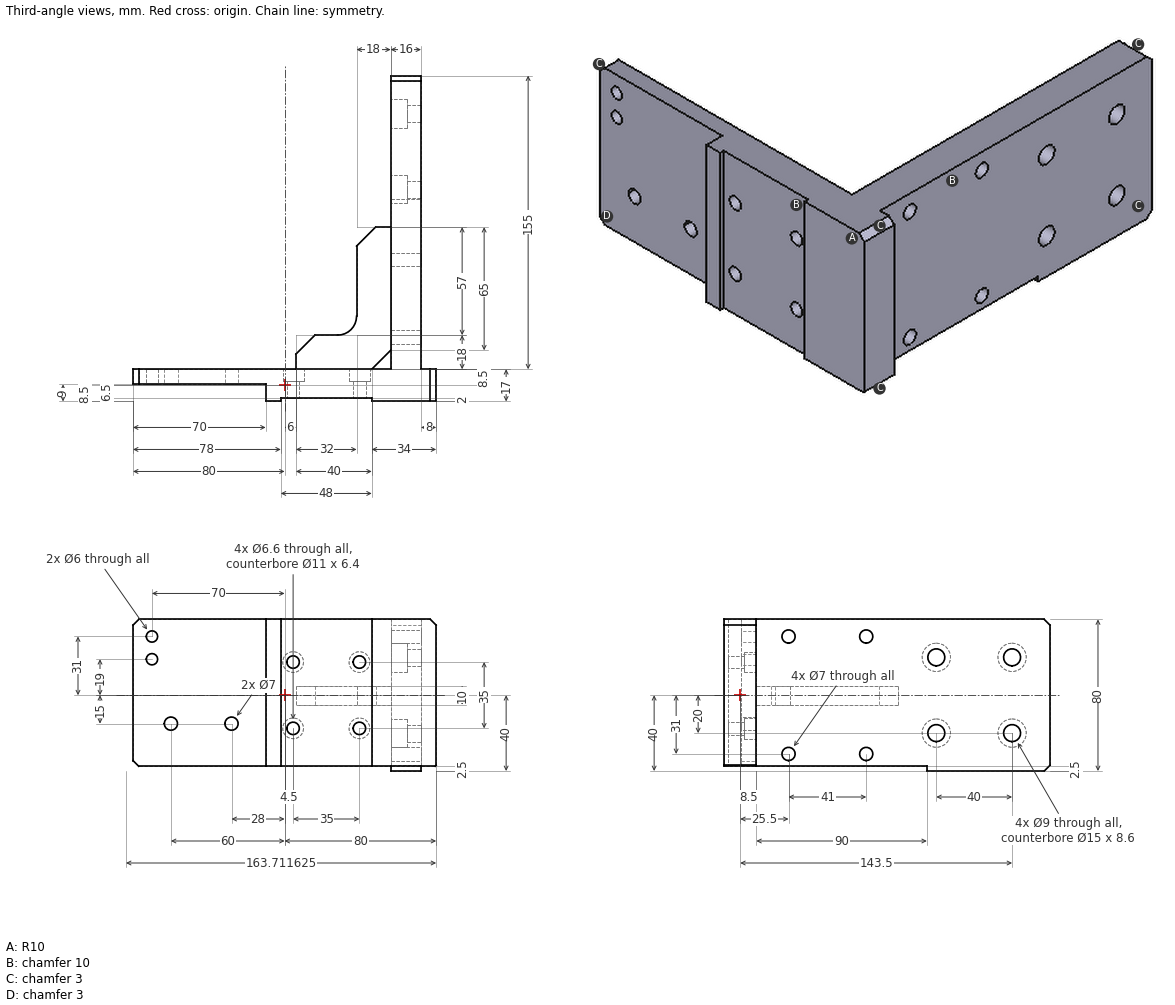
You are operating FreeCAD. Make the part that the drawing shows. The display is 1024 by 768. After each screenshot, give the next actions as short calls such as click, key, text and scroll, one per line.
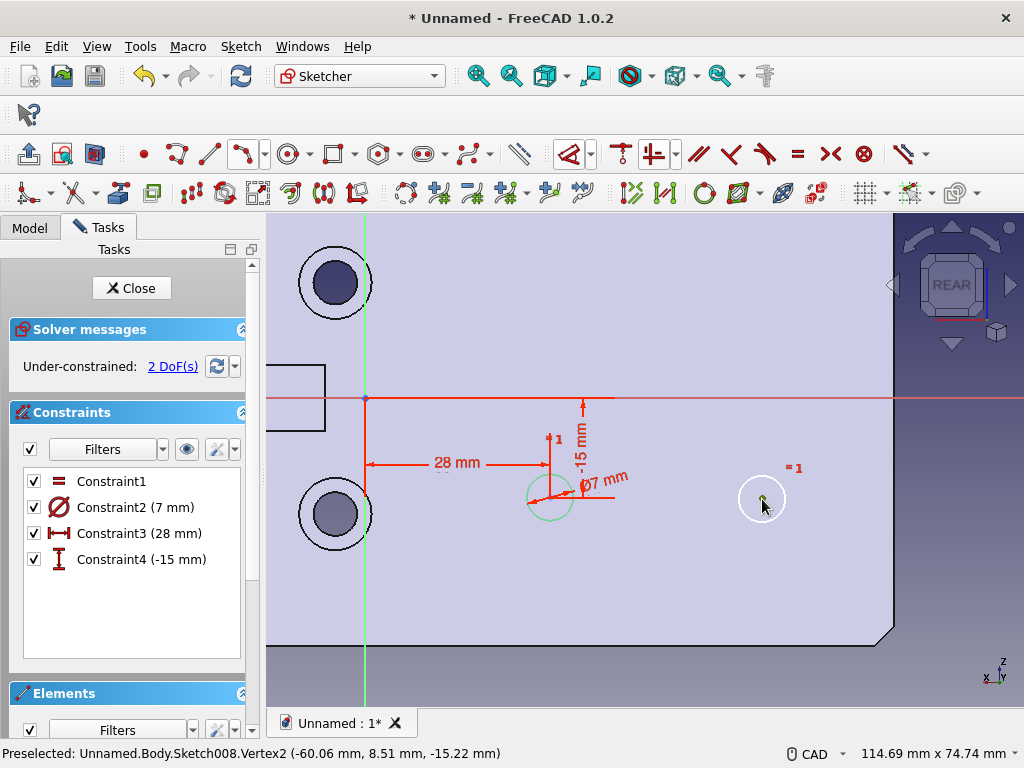
click(590, 154)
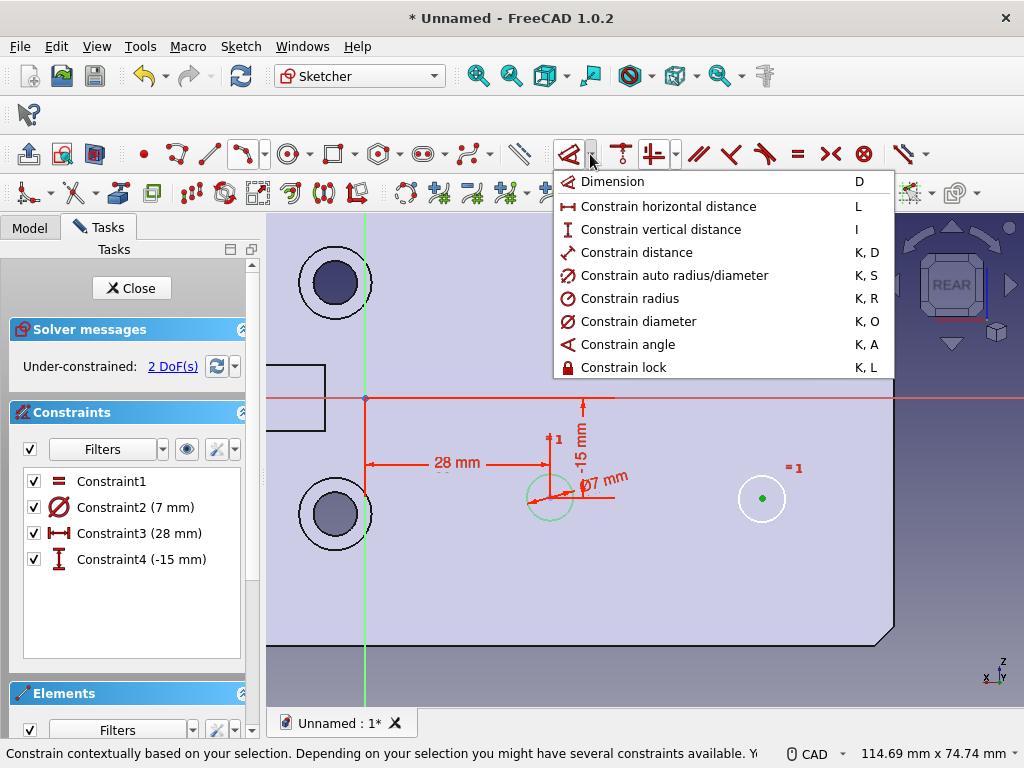
click(724, 206)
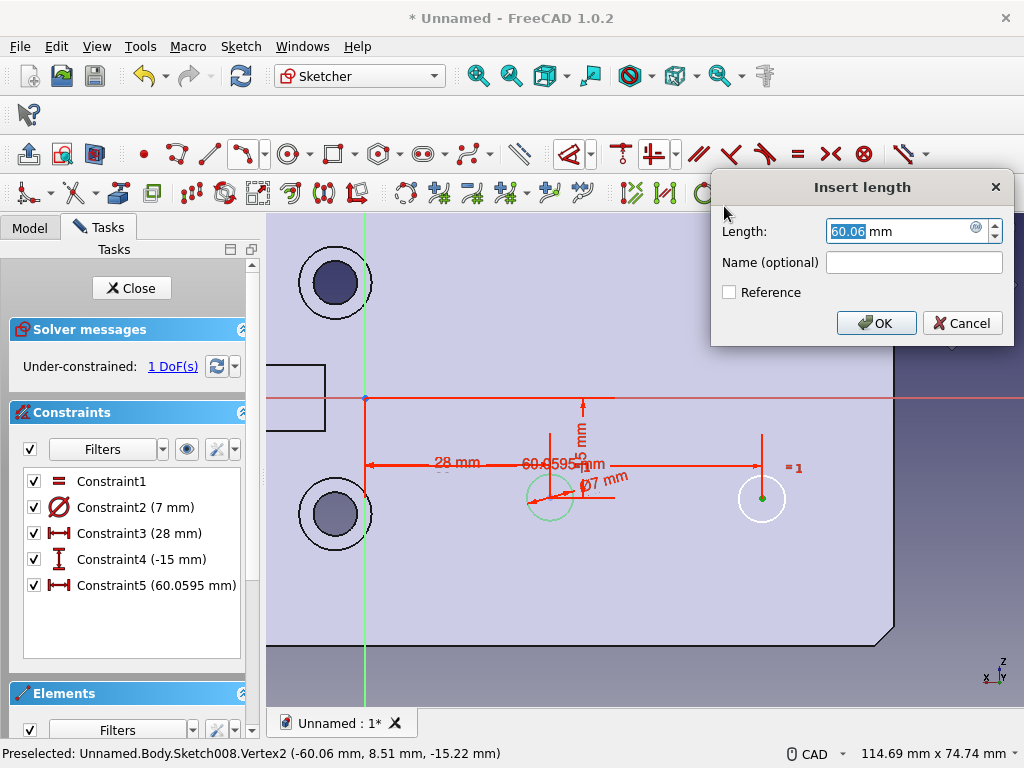
text(60)
key(Return)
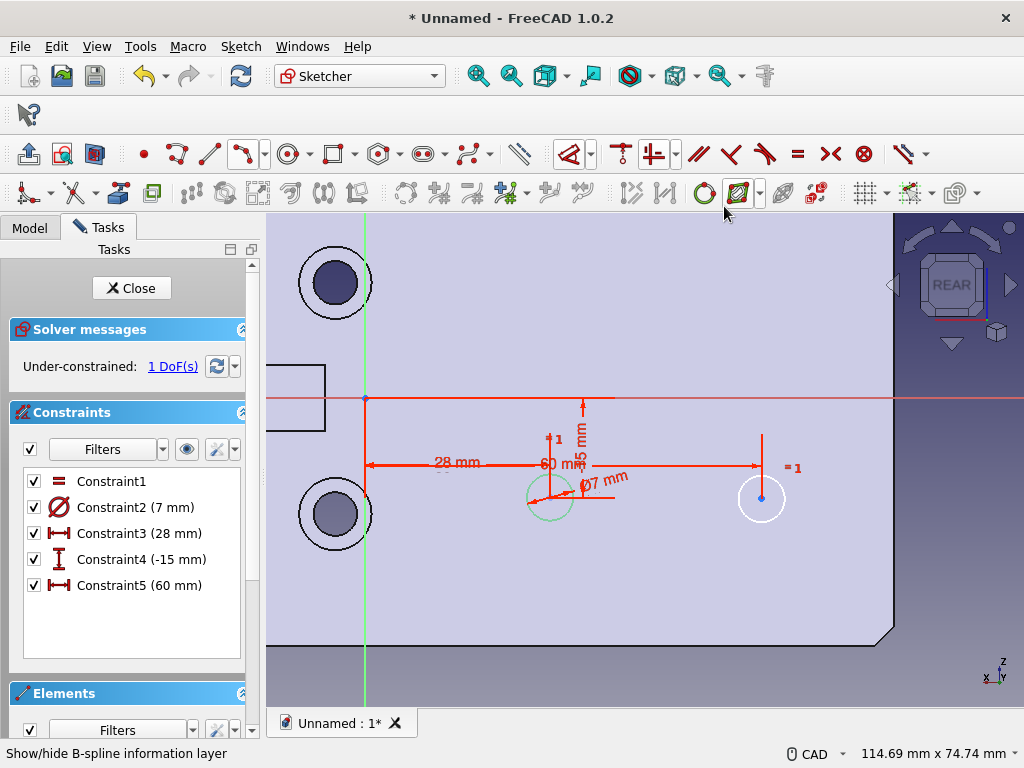
click(762, 499)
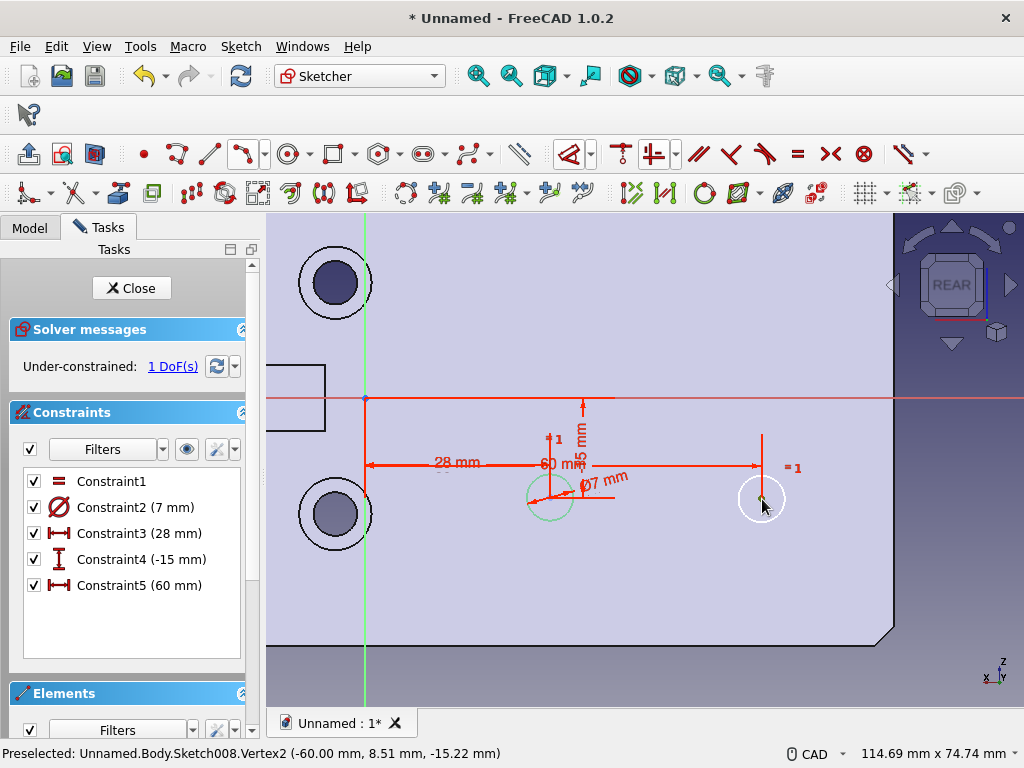
key(i)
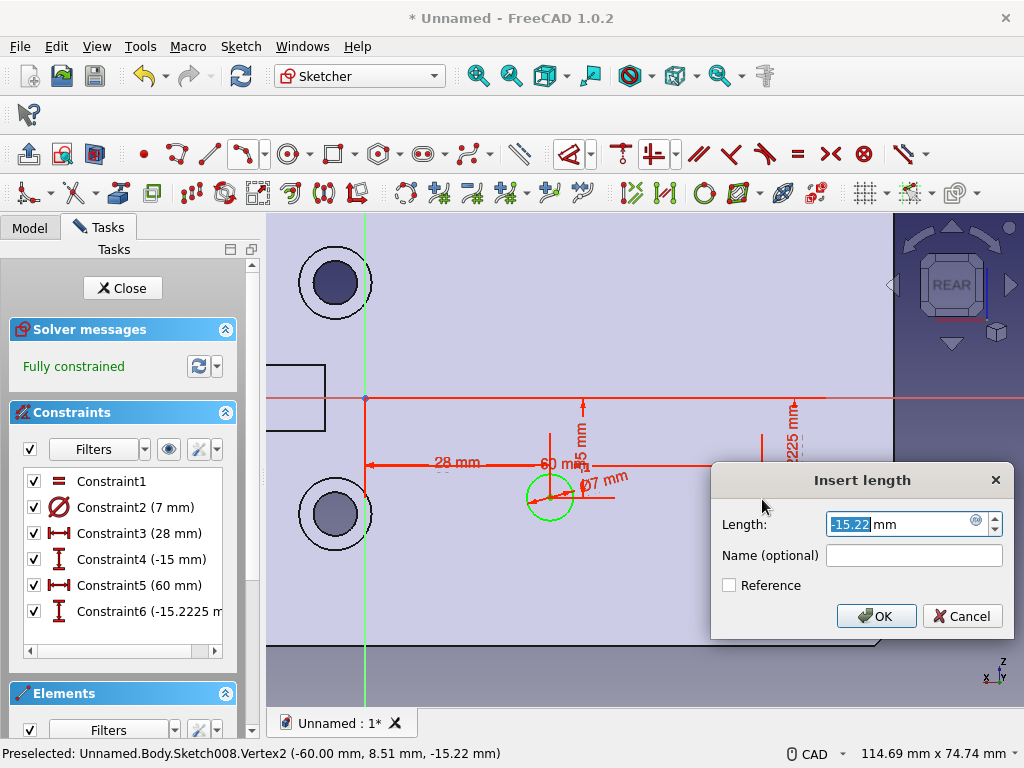
text(-15)
key(Return)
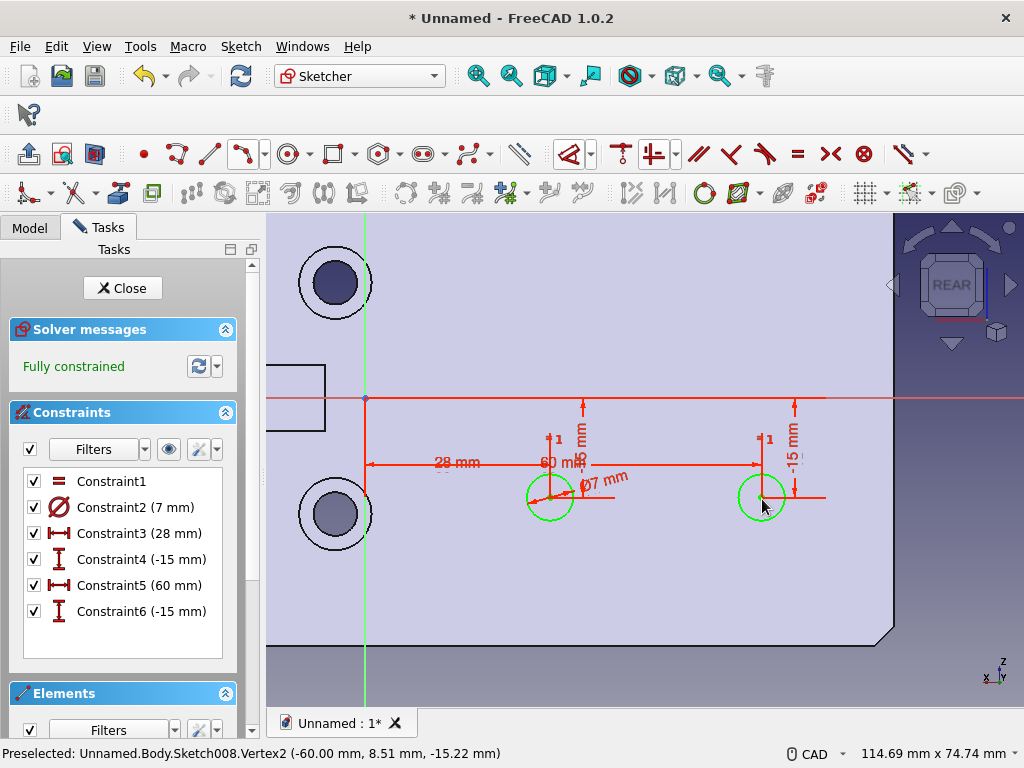
click(123, 288)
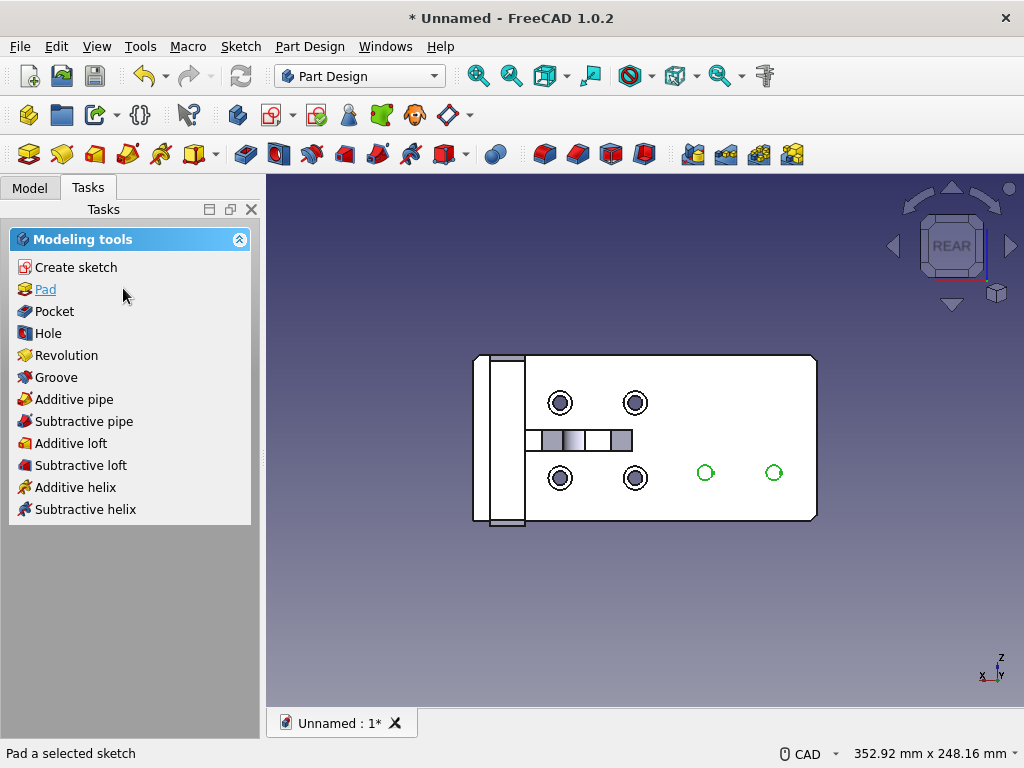
click(246, 154)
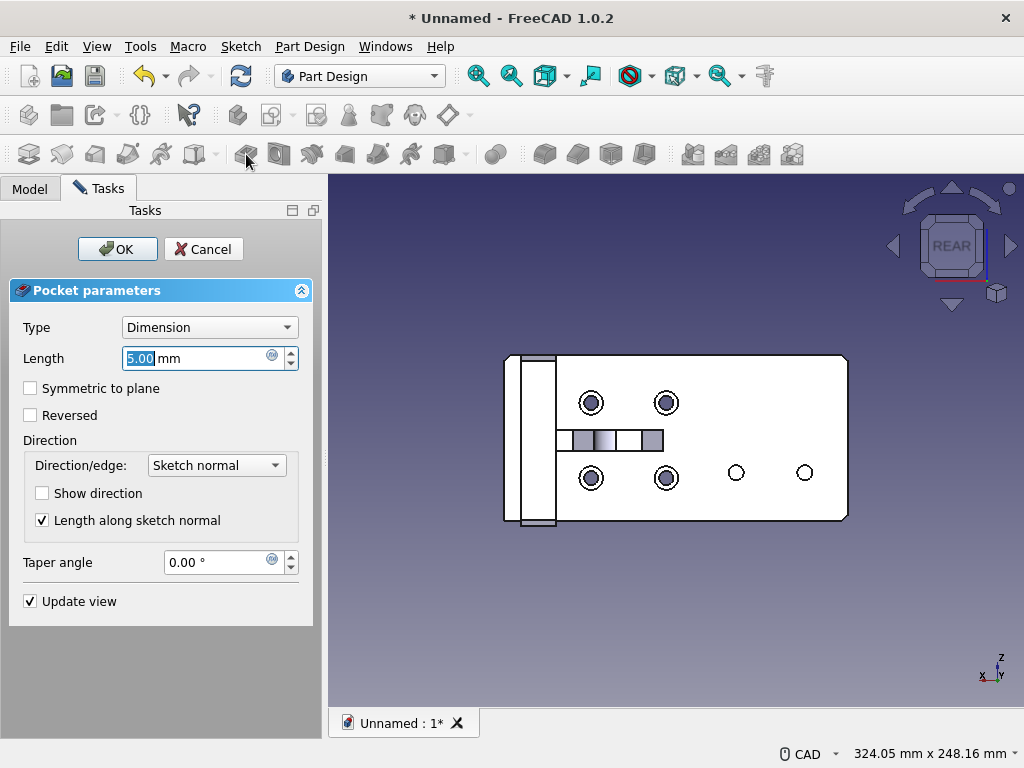
click(210, 328)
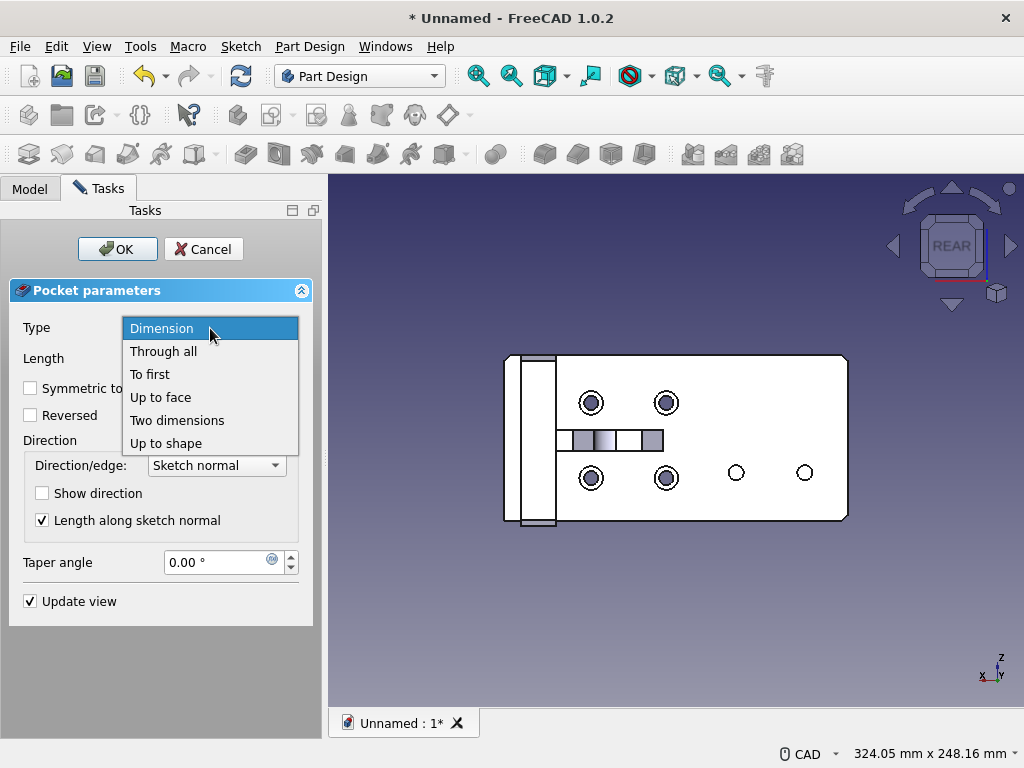
click(208, 352)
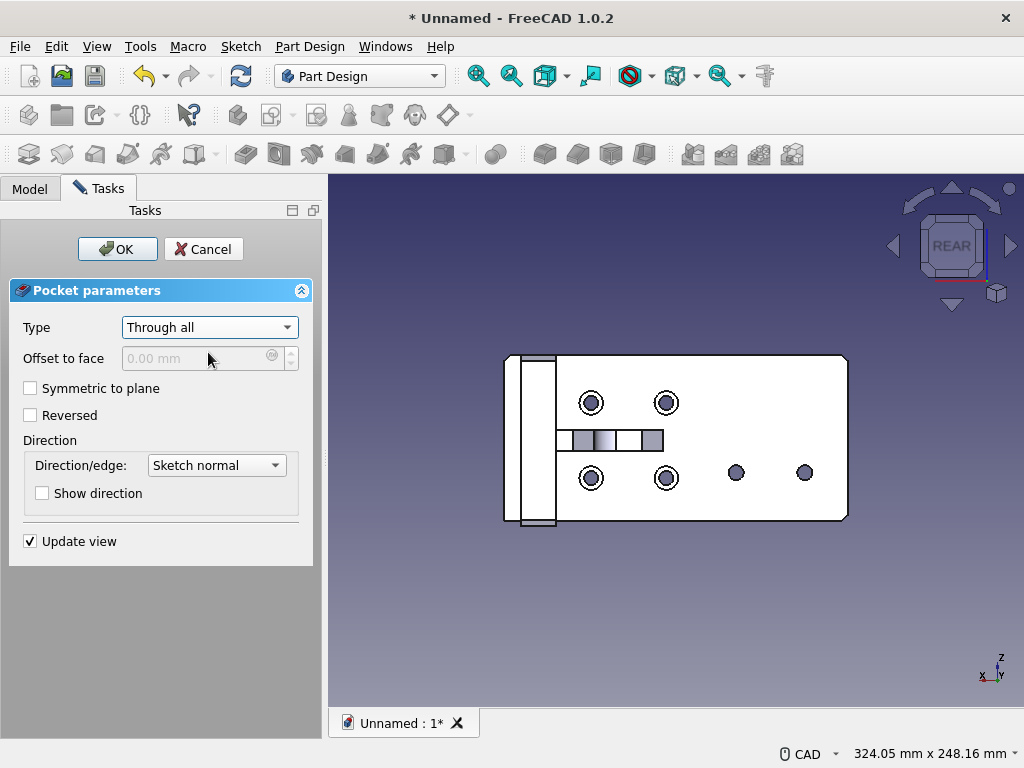
click(118, 249)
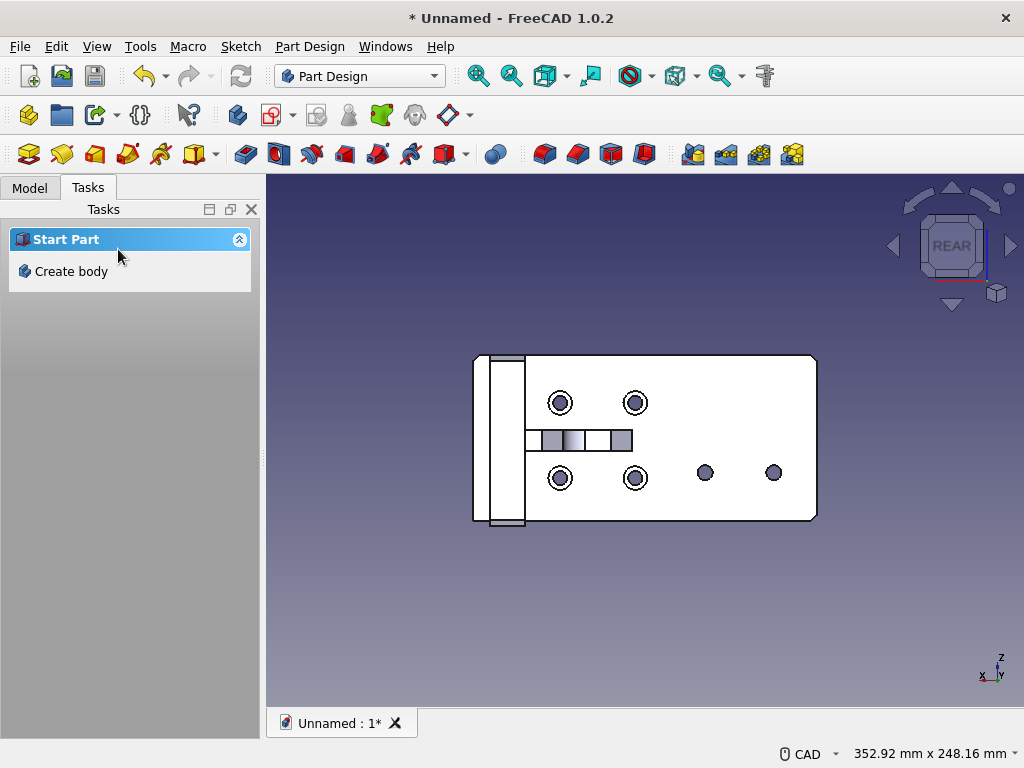
click(754, 413)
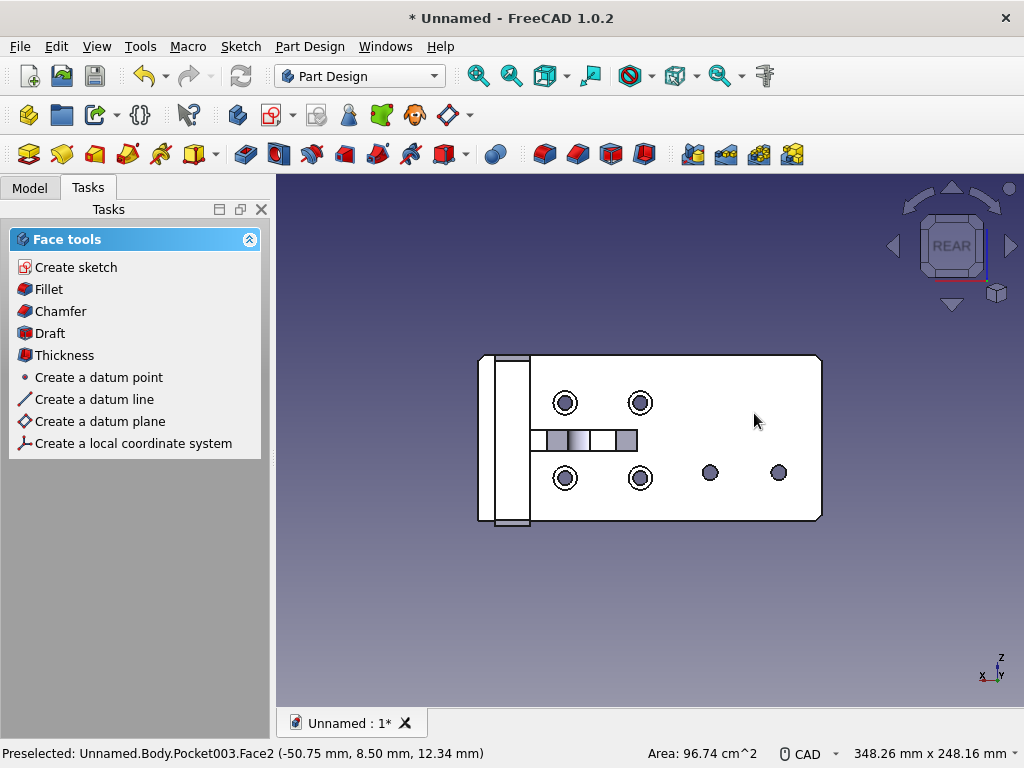
click(270, 116)